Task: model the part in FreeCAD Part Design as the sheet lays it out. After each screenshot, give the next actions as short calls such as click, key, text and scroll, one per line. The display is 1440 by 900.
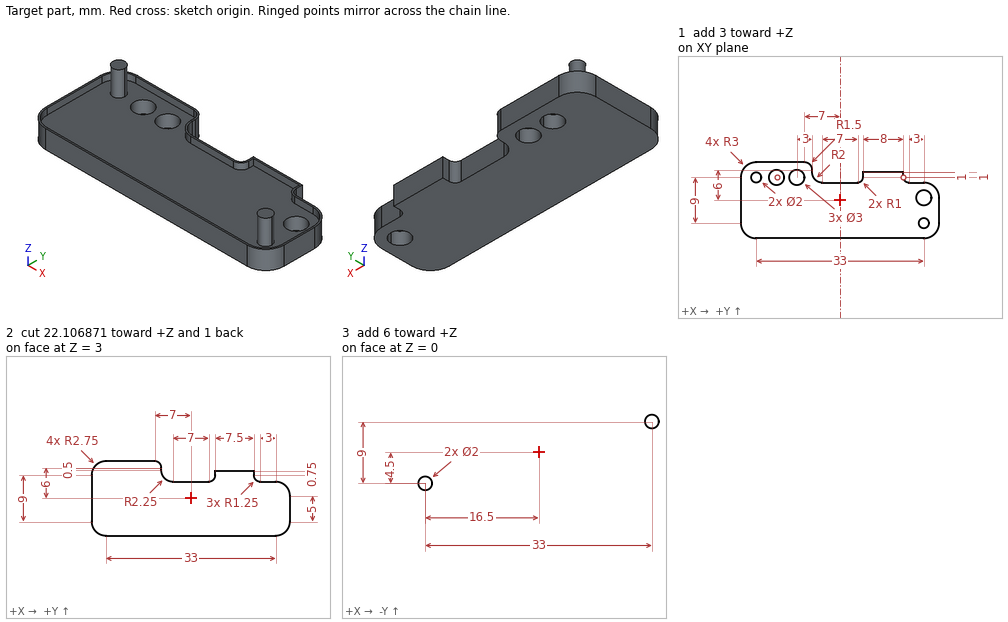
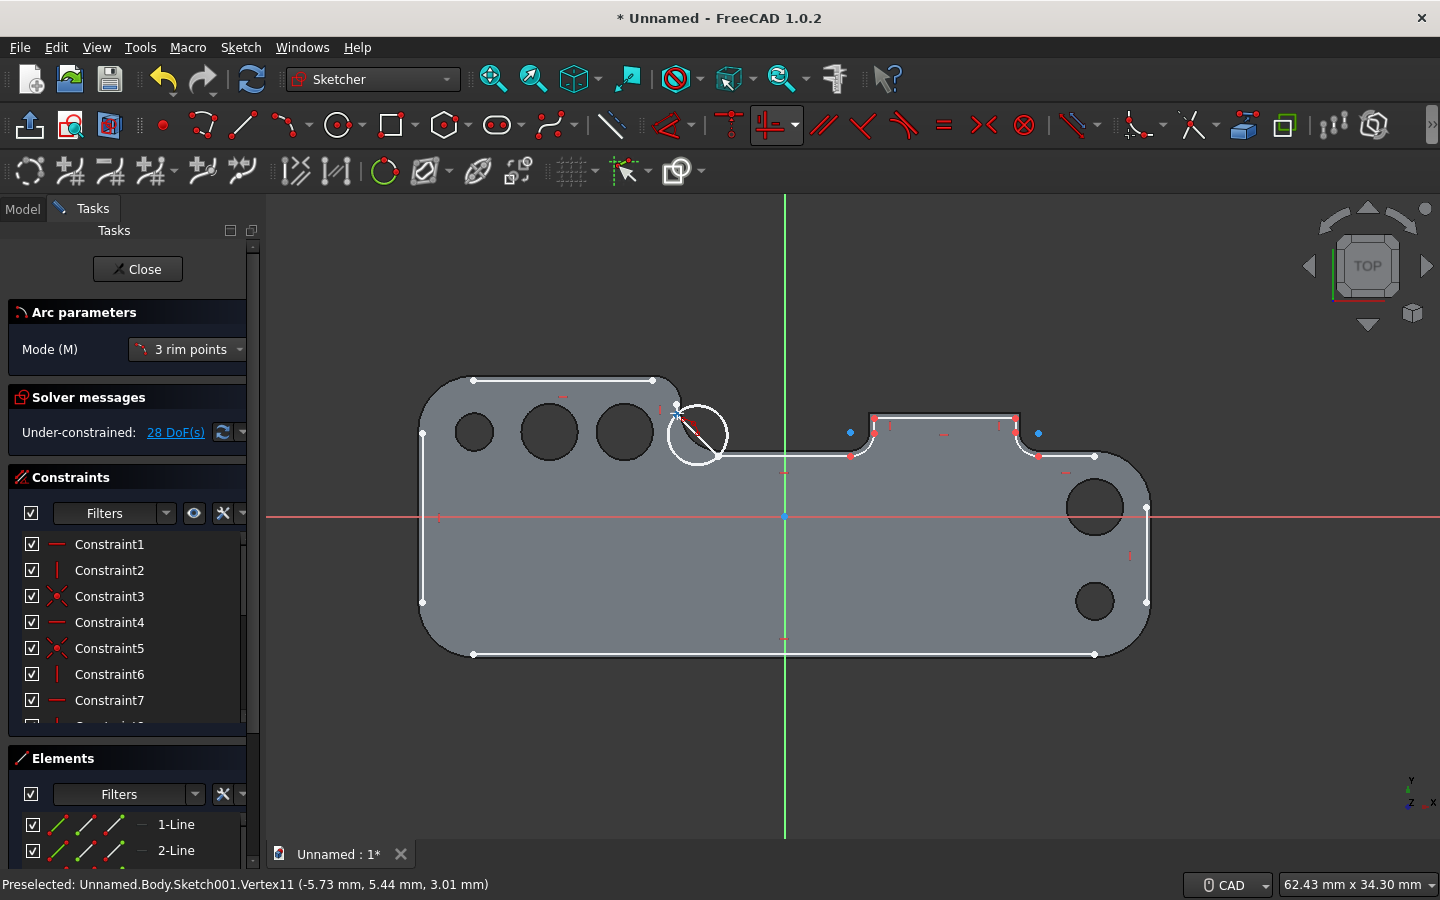
scroll(689, 443, up, 2)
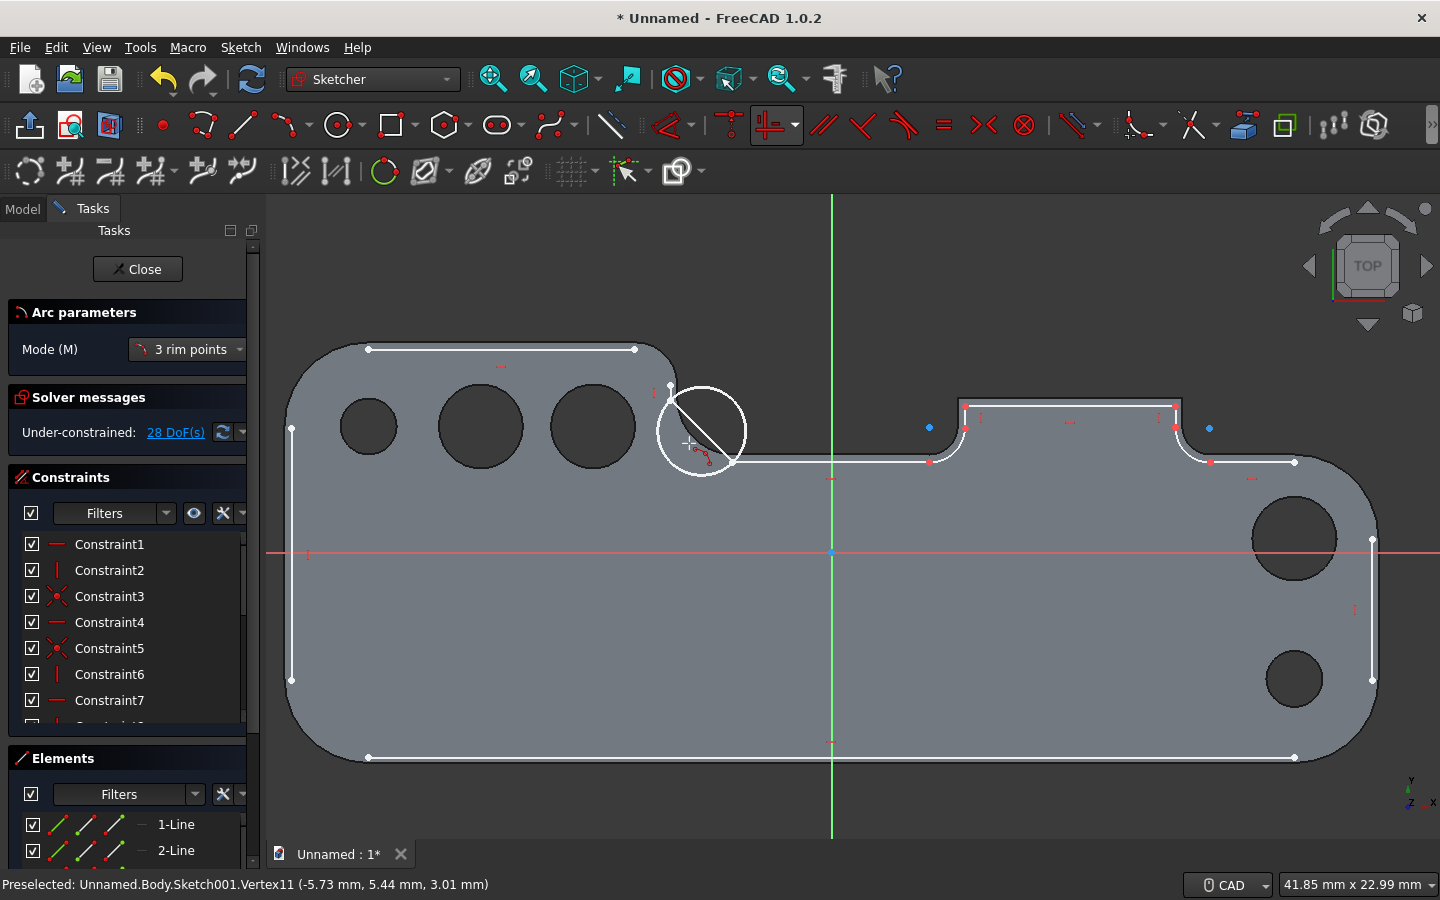
click(689, 443)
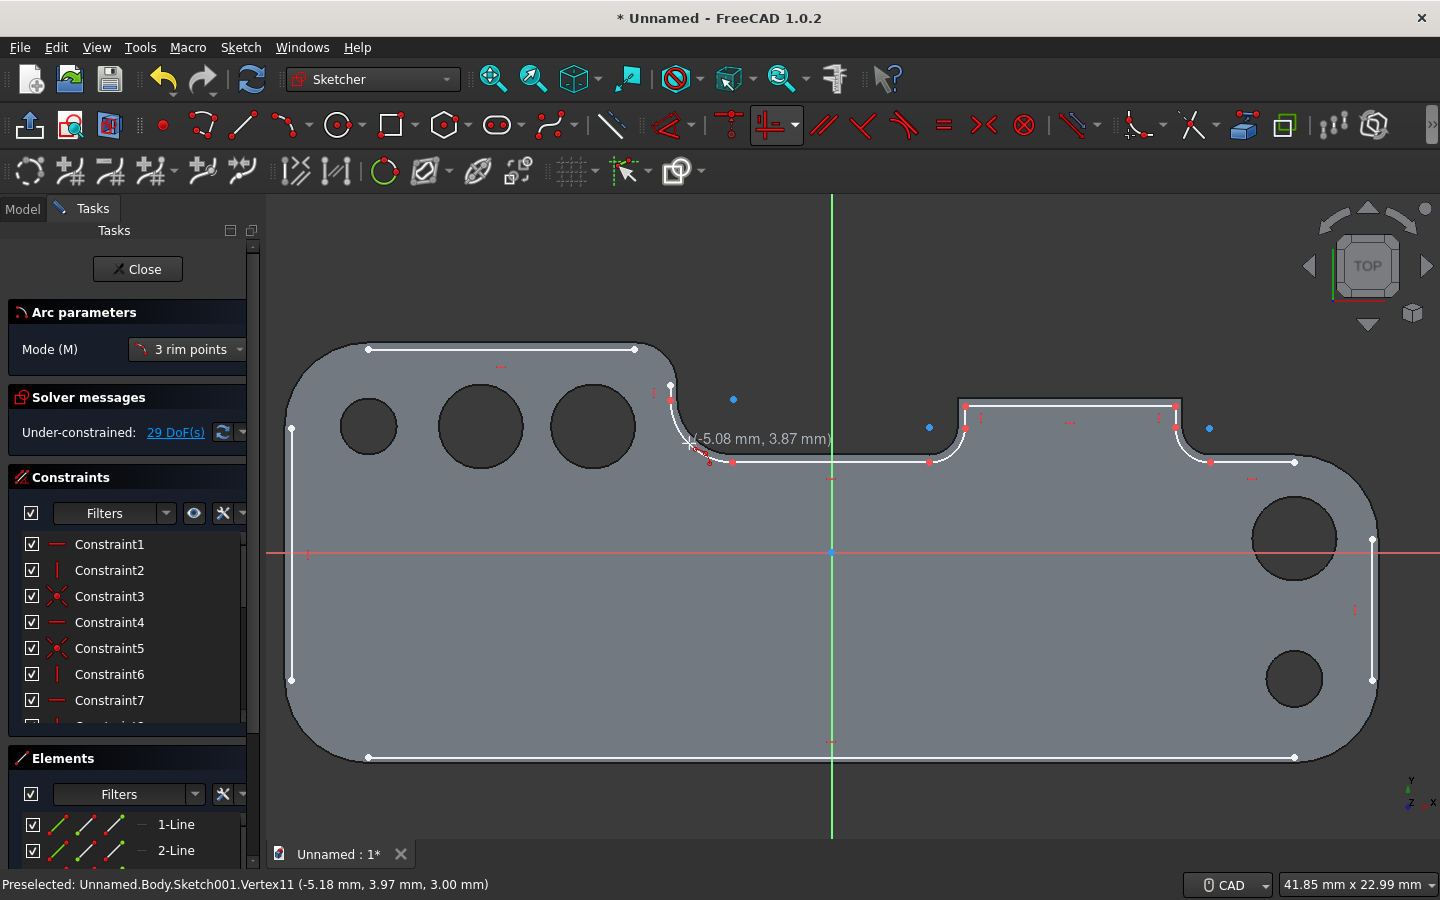
scroll(670, 384, up, 5)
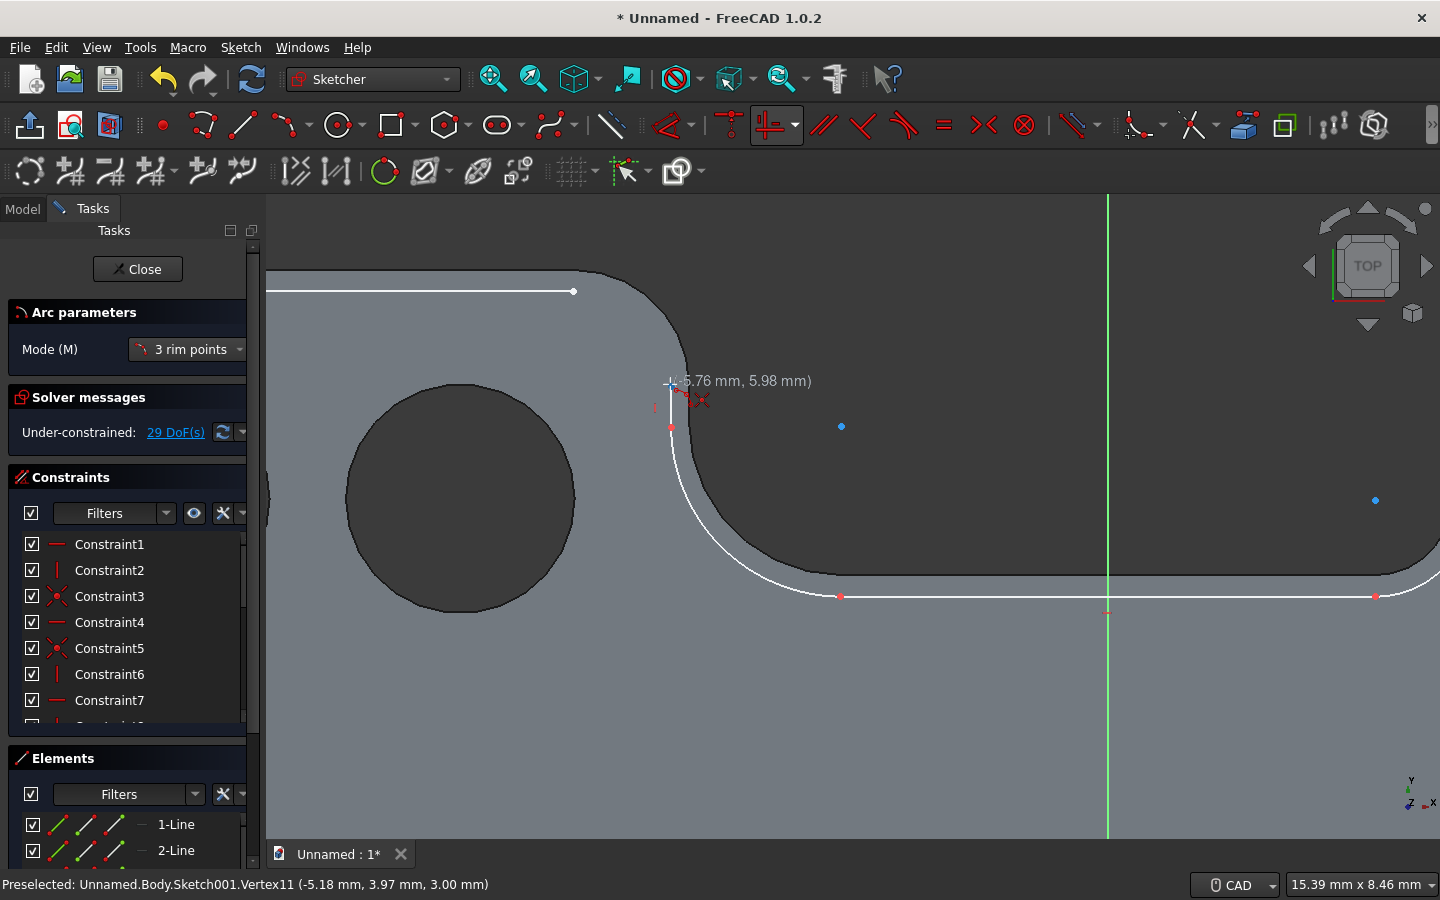
click(671, 387)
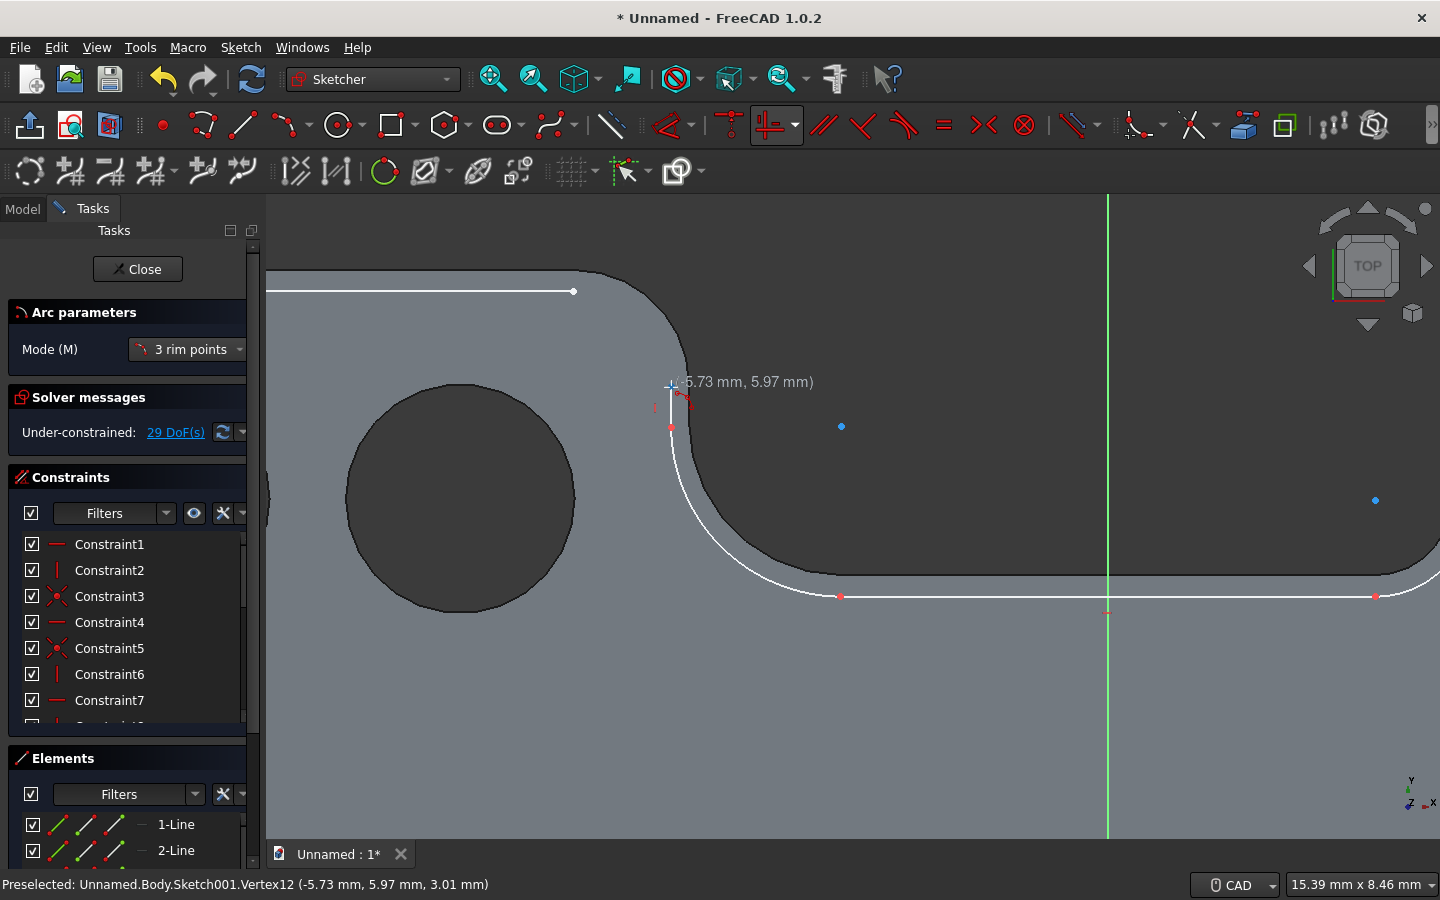
scroll(678, 410, down, 7)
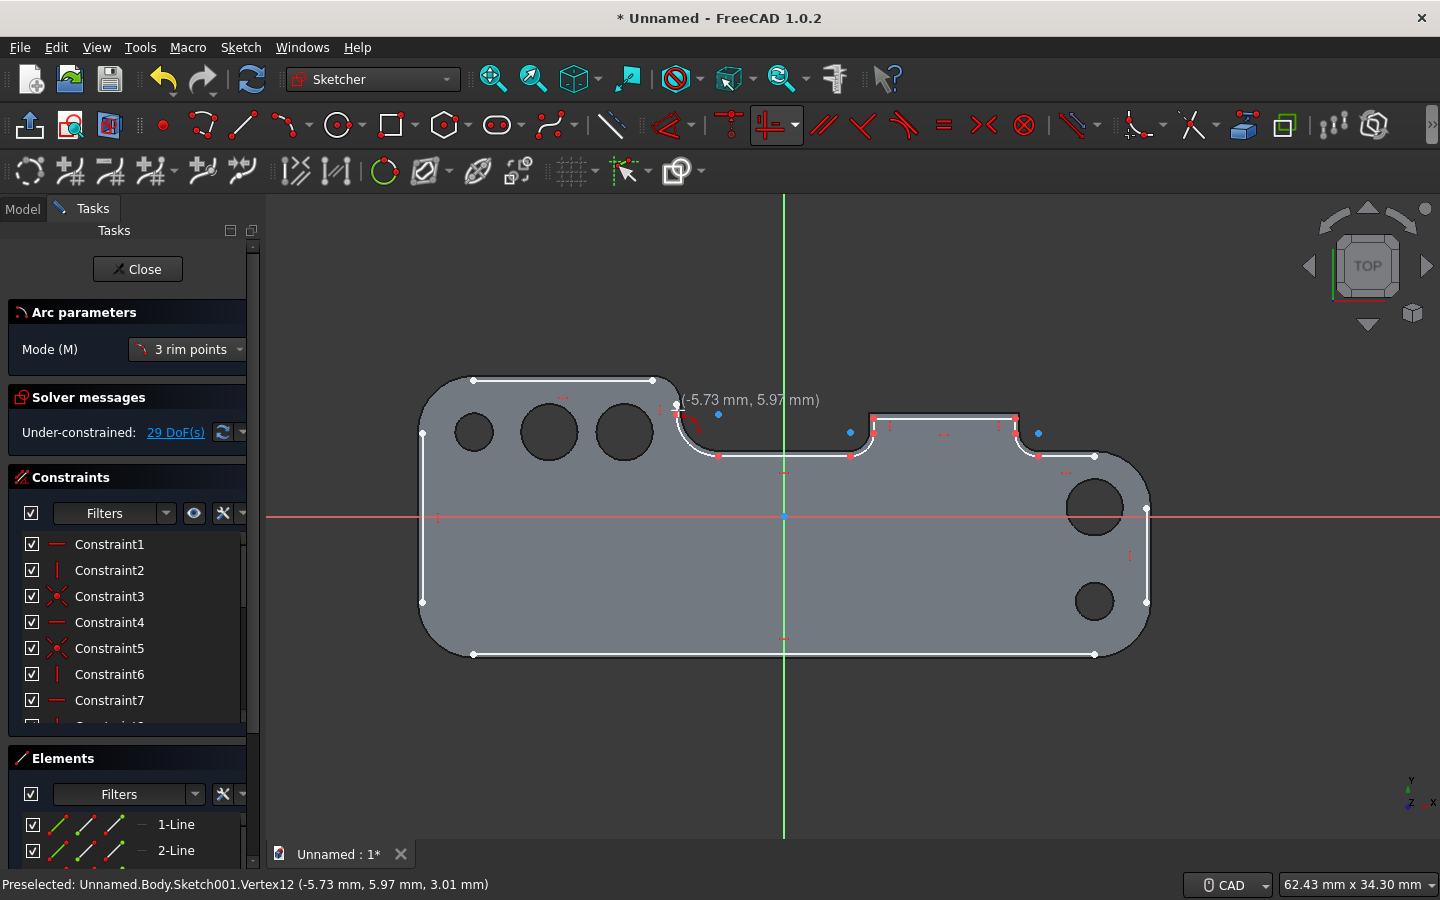
click(653, 381)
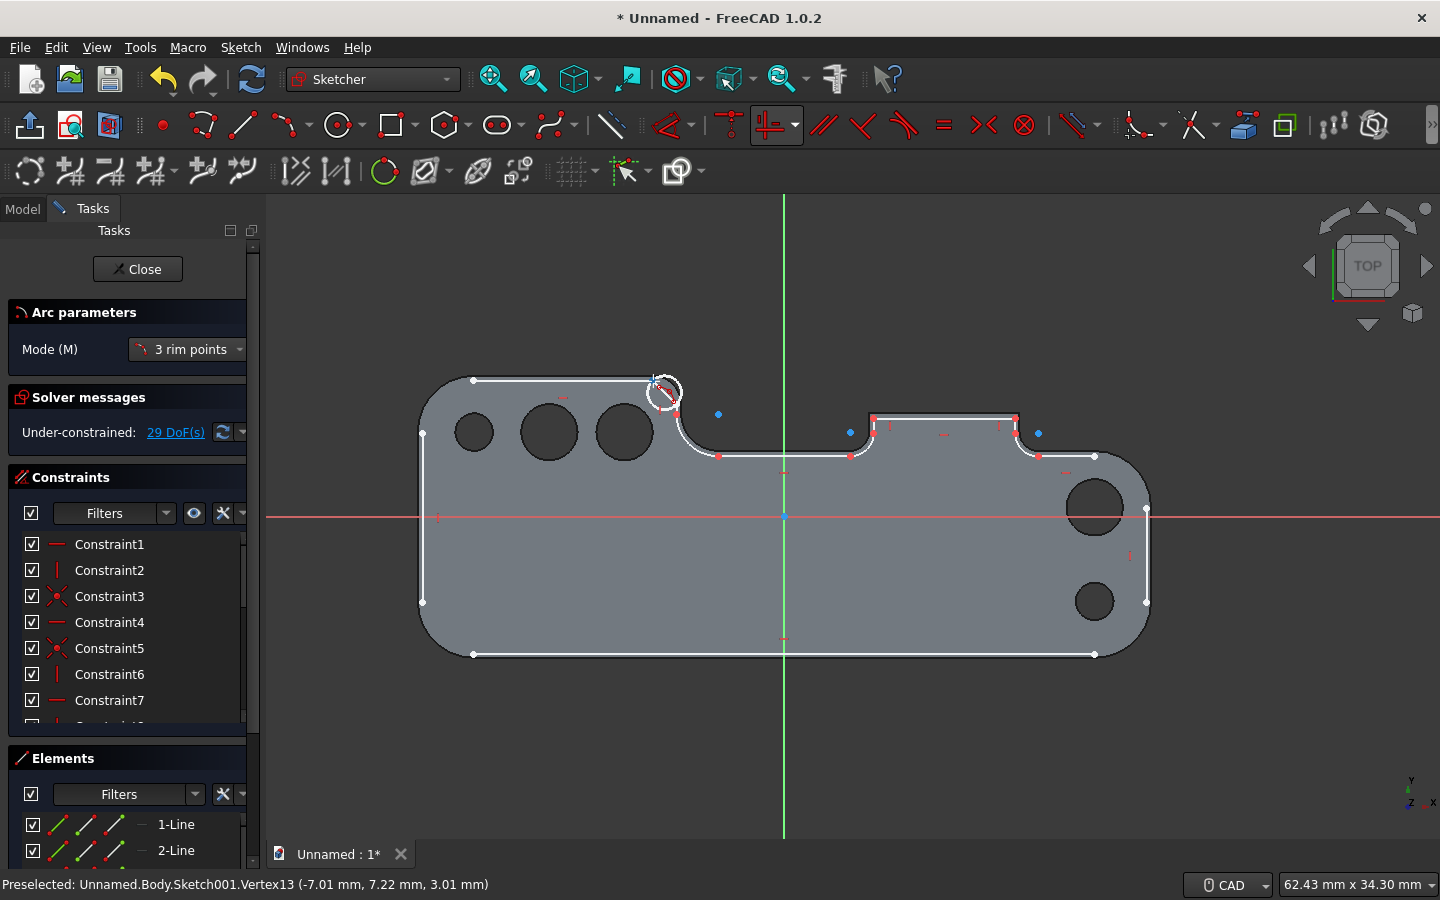
scroll(669, 387, up, 5)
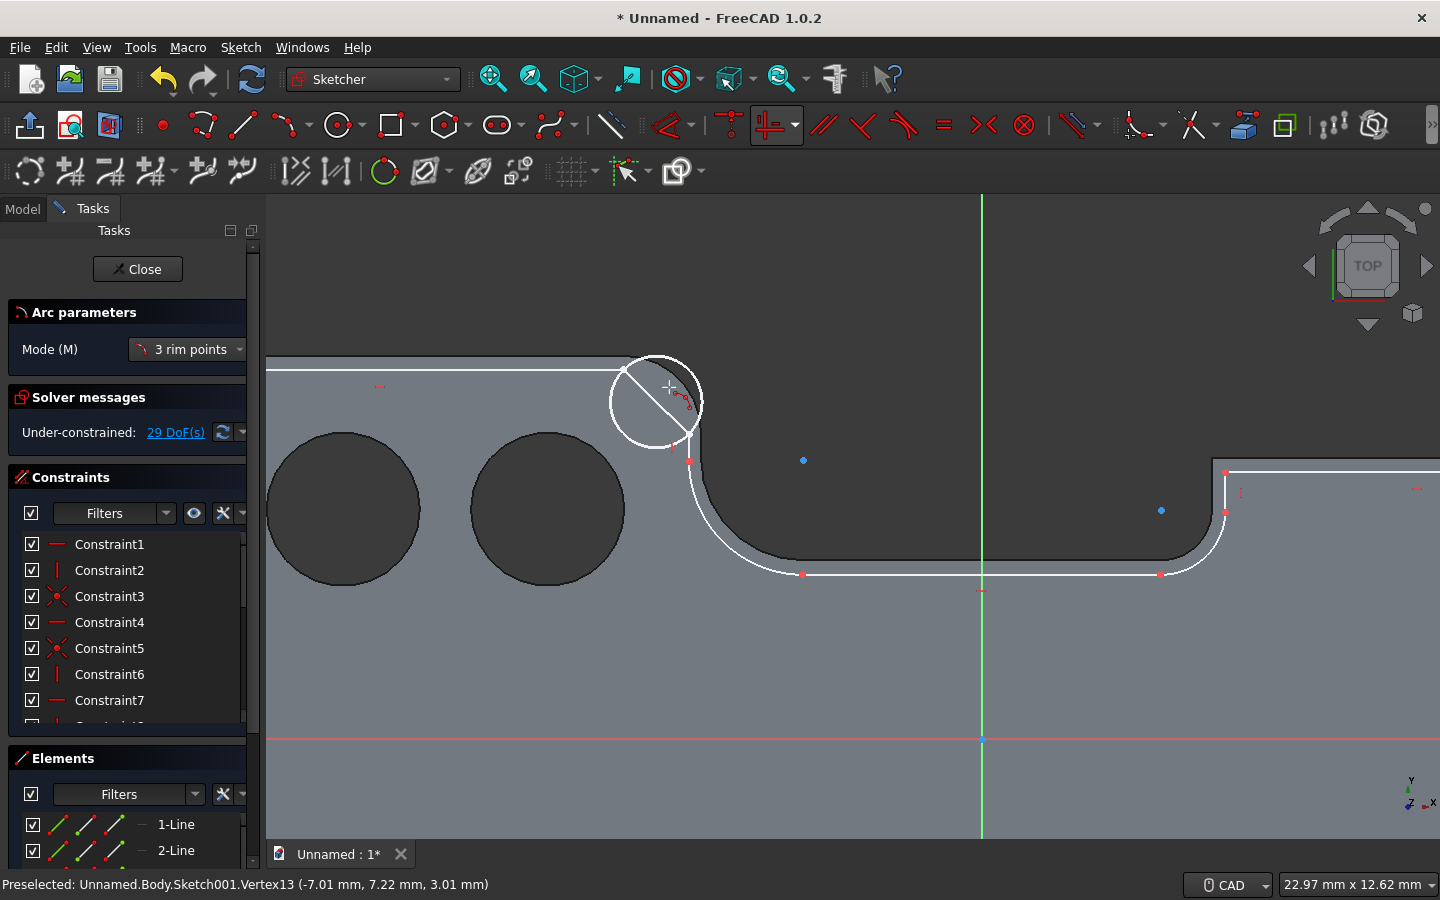
click(670, 387)